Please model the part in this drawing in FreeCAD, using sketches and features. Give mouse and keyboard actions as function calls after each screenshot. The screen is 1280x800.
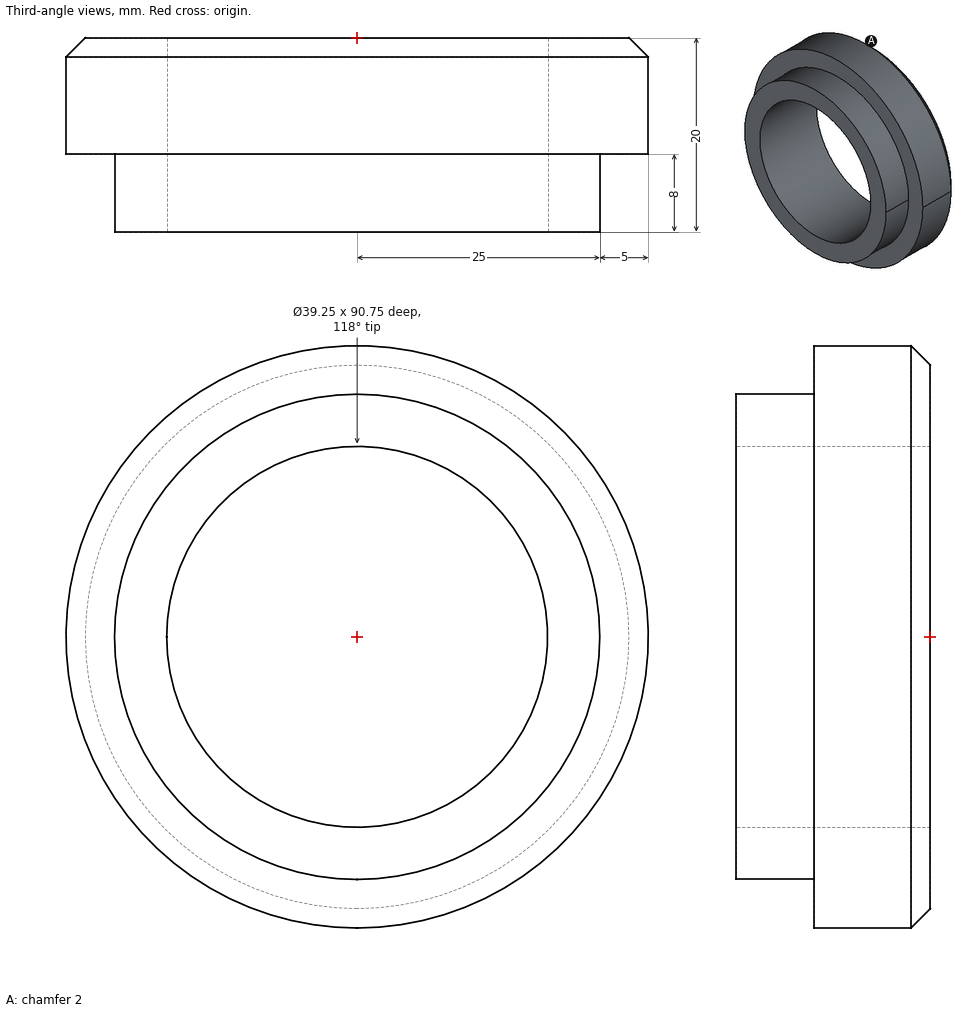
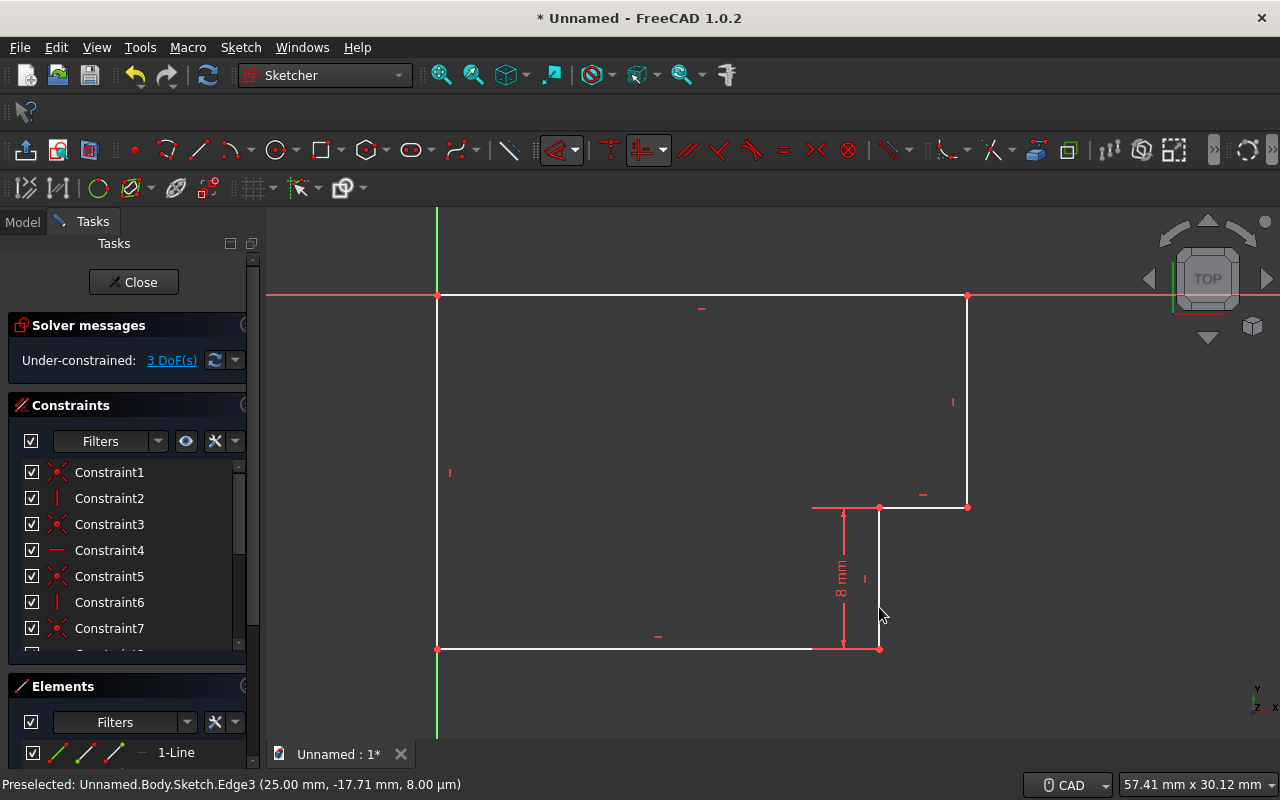
click(905, 508)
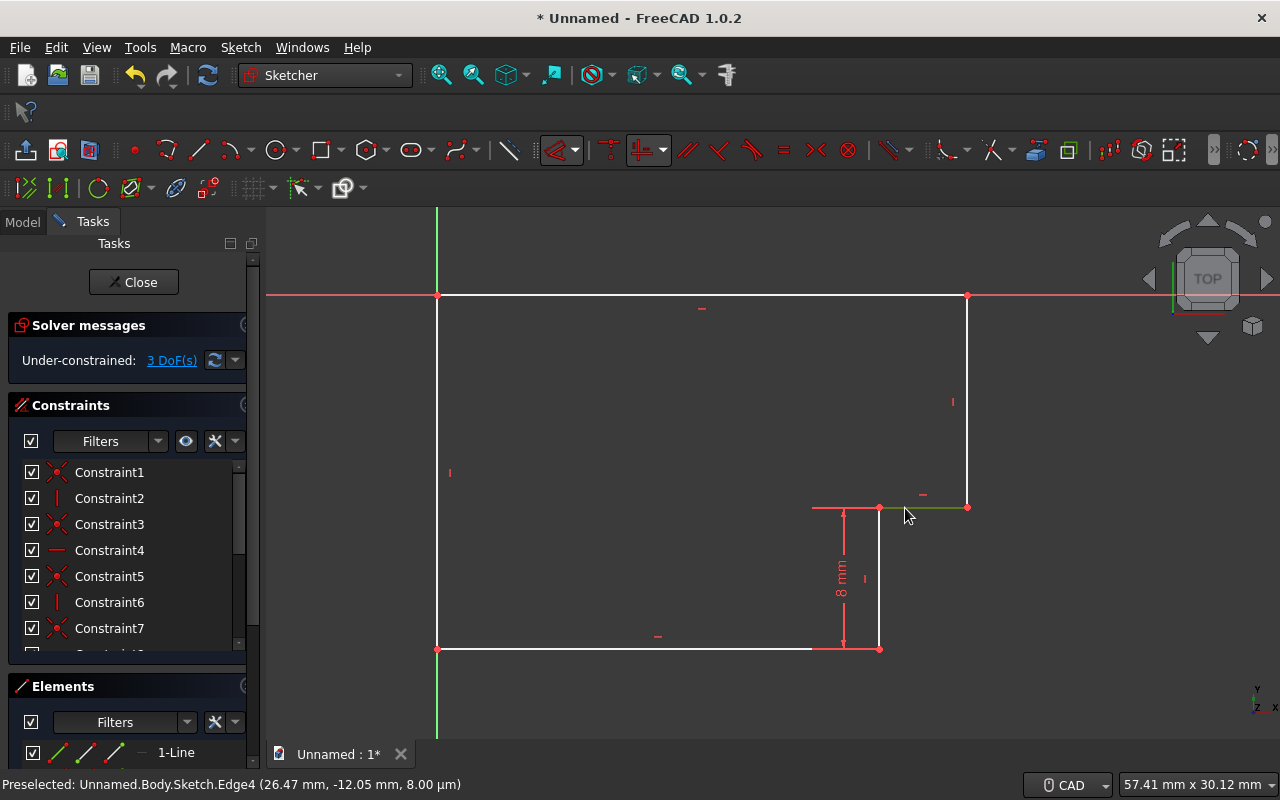
key(l)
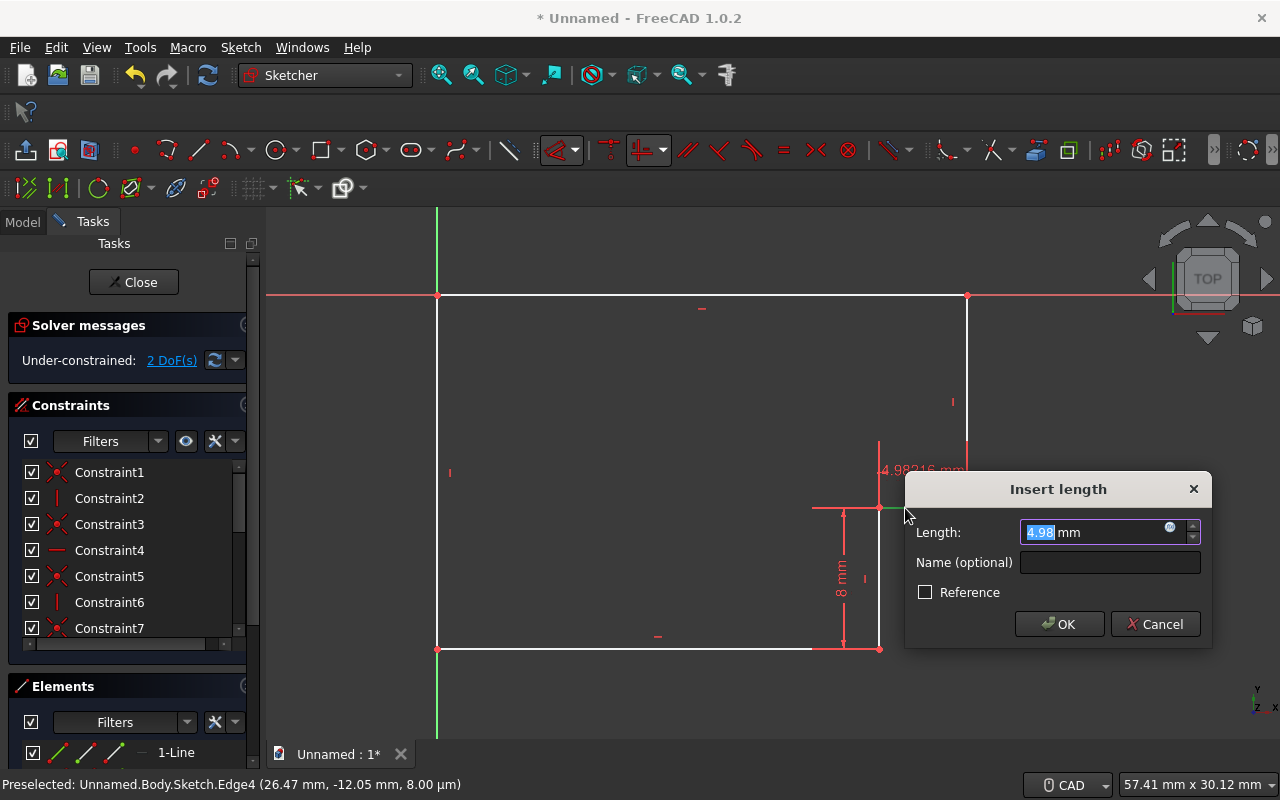
text(5)
key(Return)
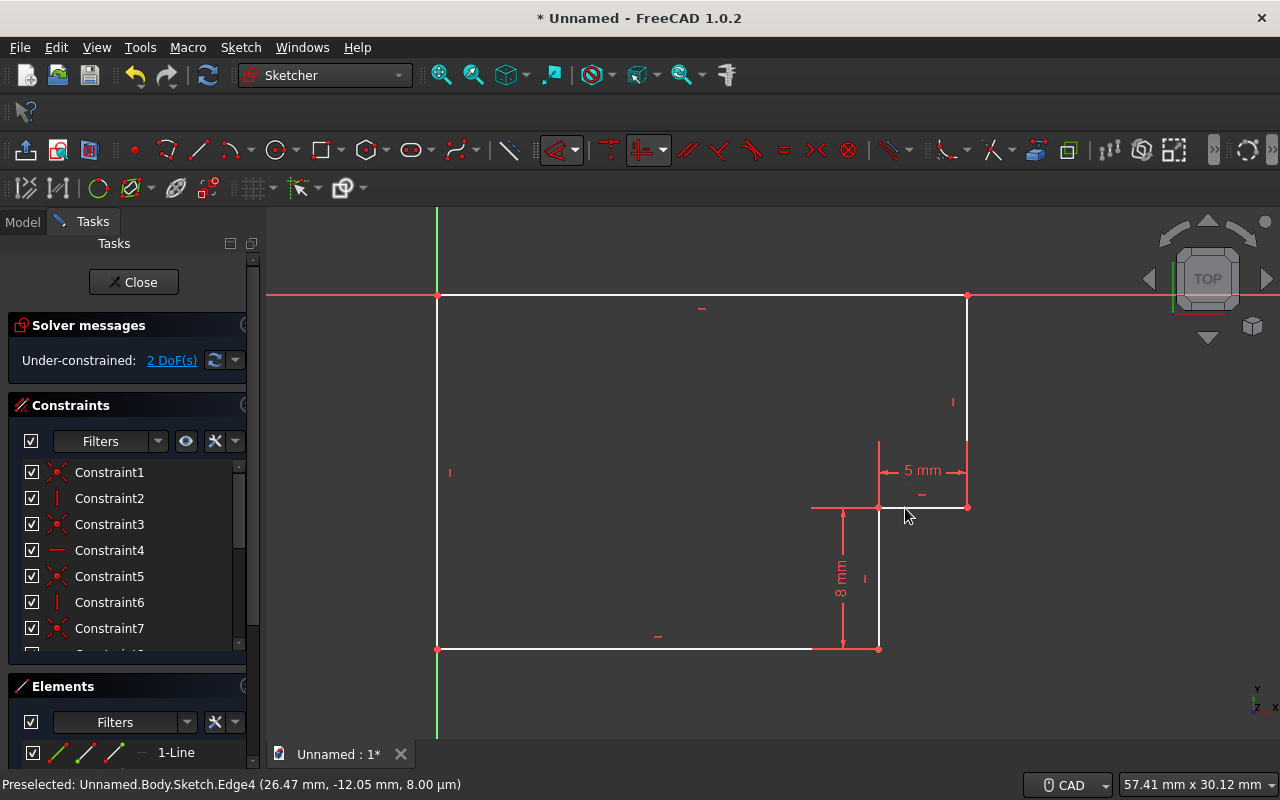
click(437, 401)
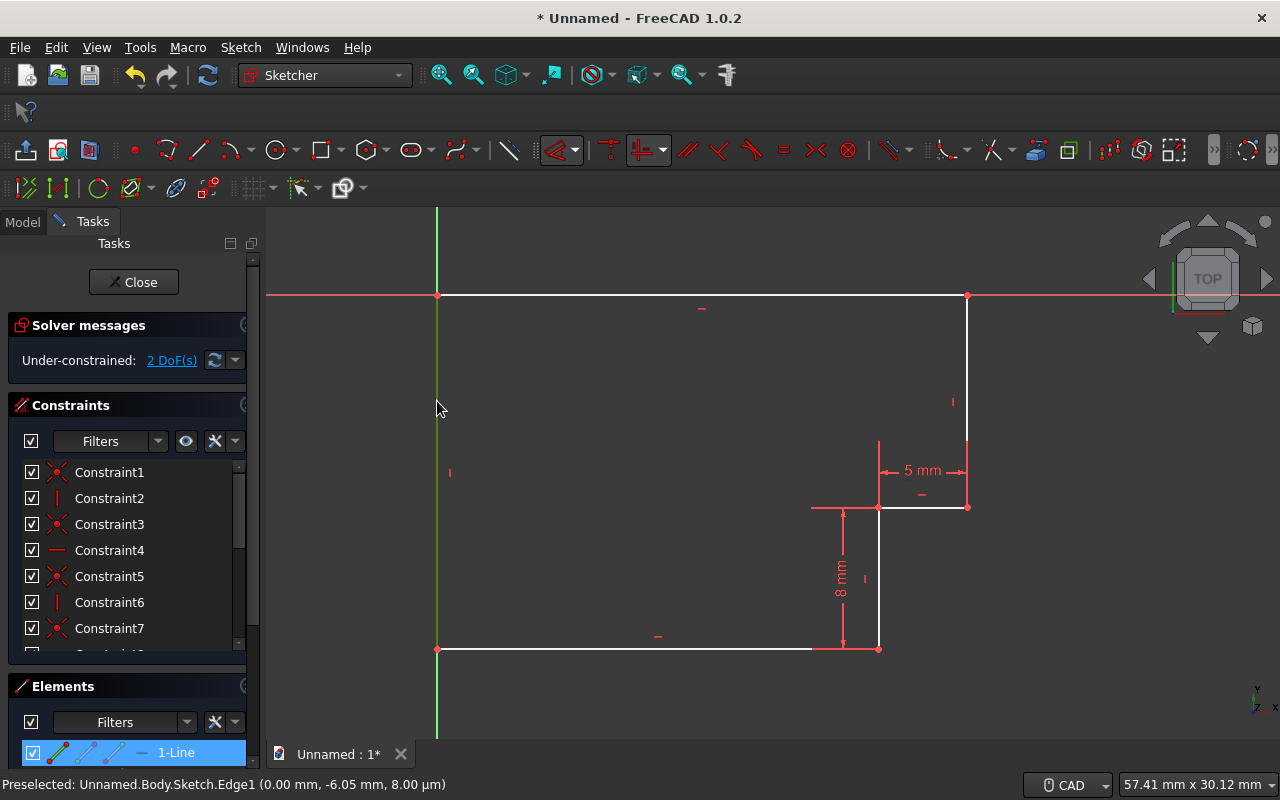
click(578, 150)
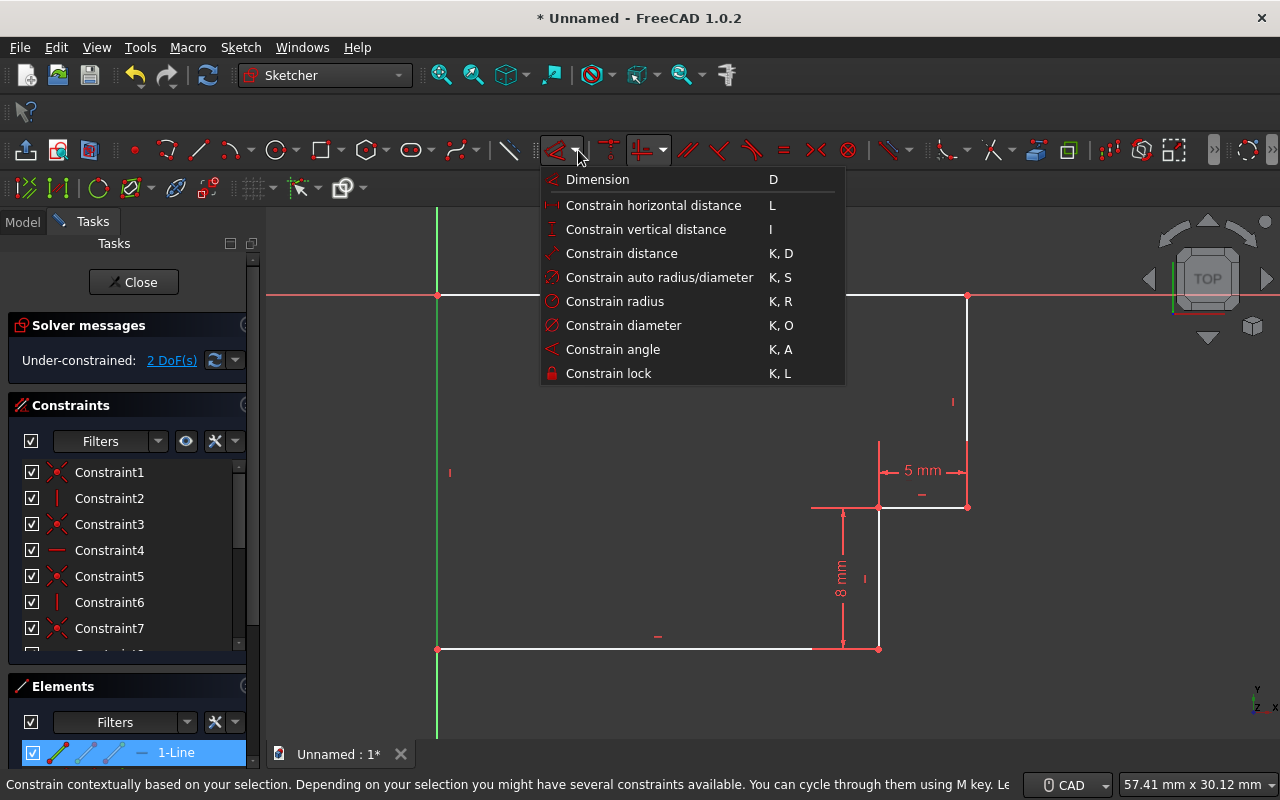
click(693, 229)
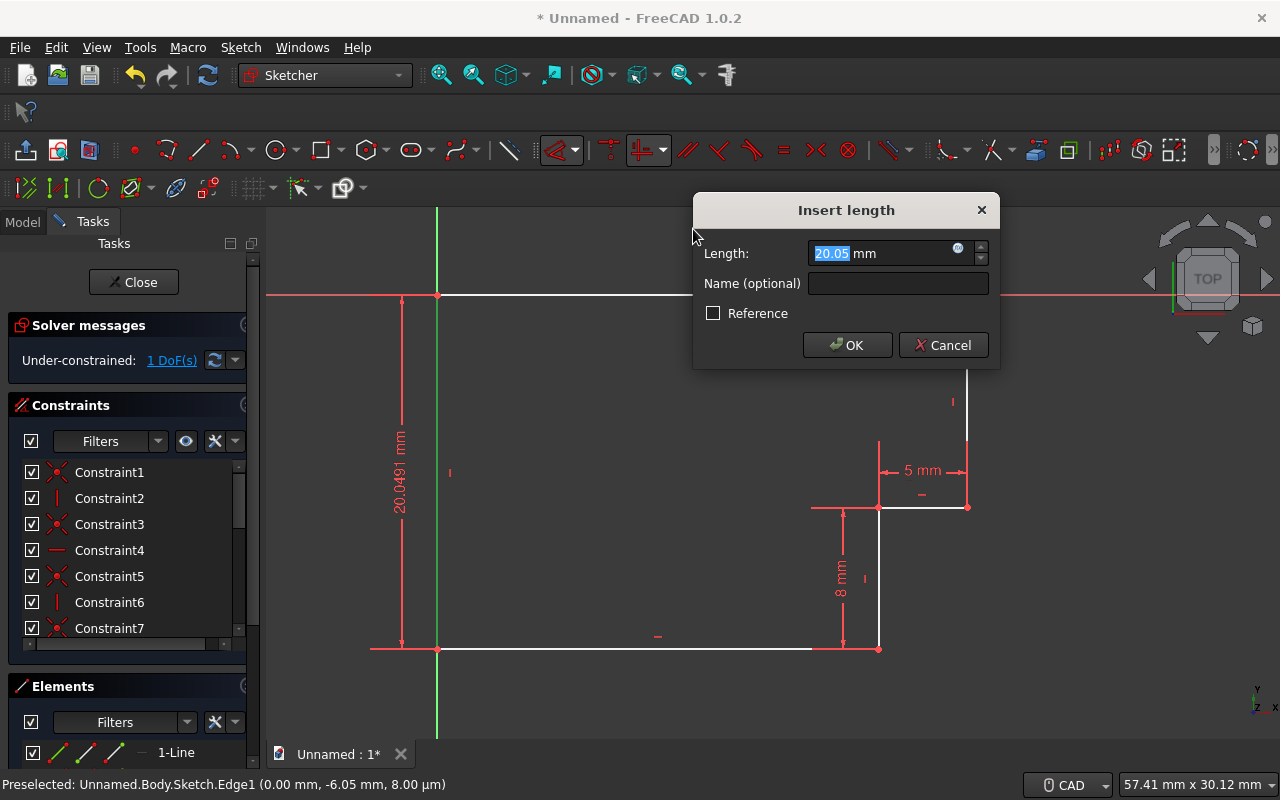
text(20)
key(Return)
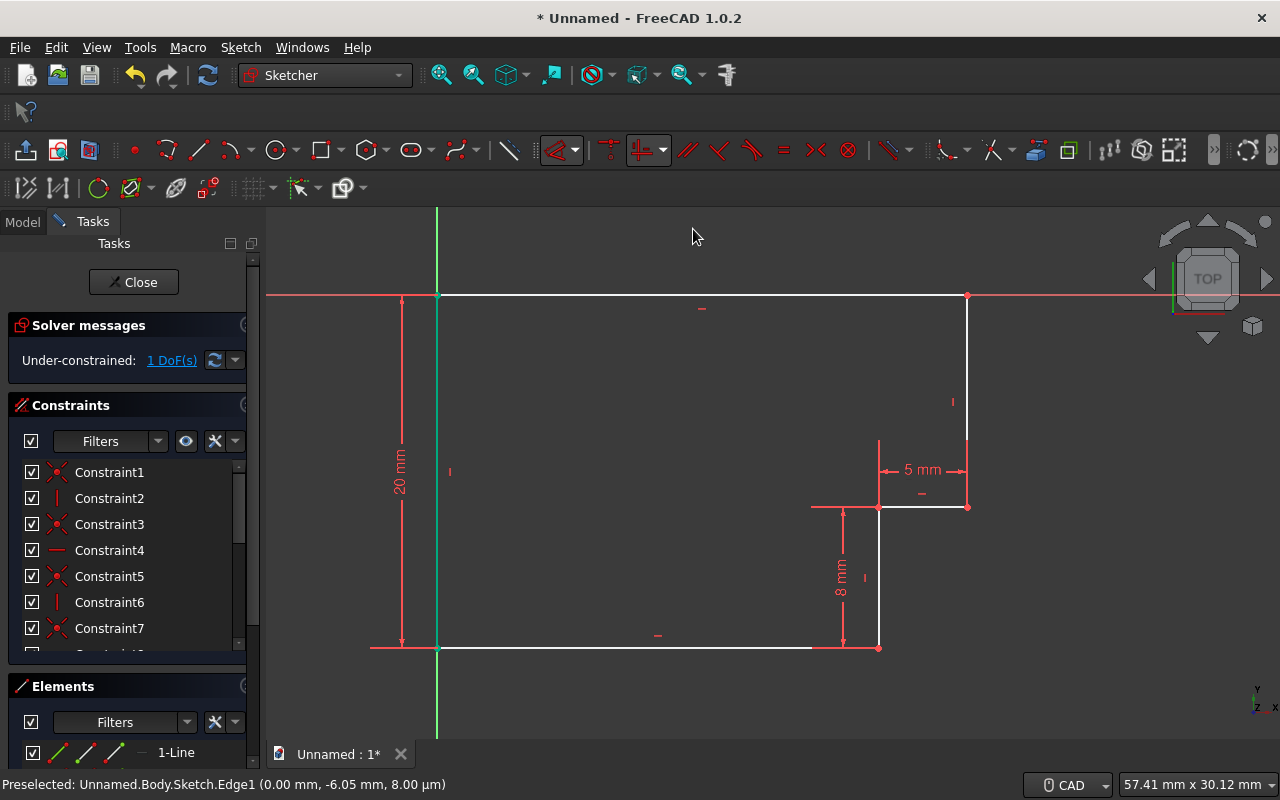
click(570, 648)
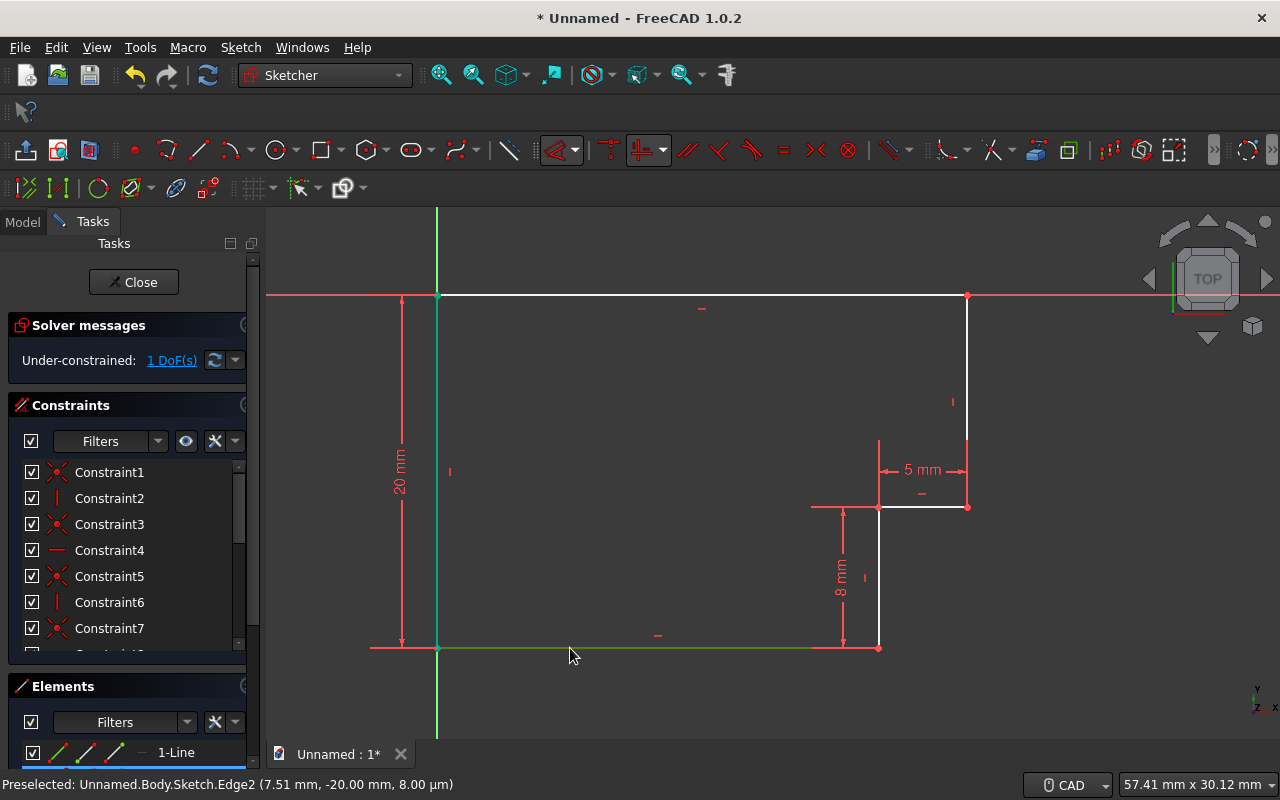
click(578, 150)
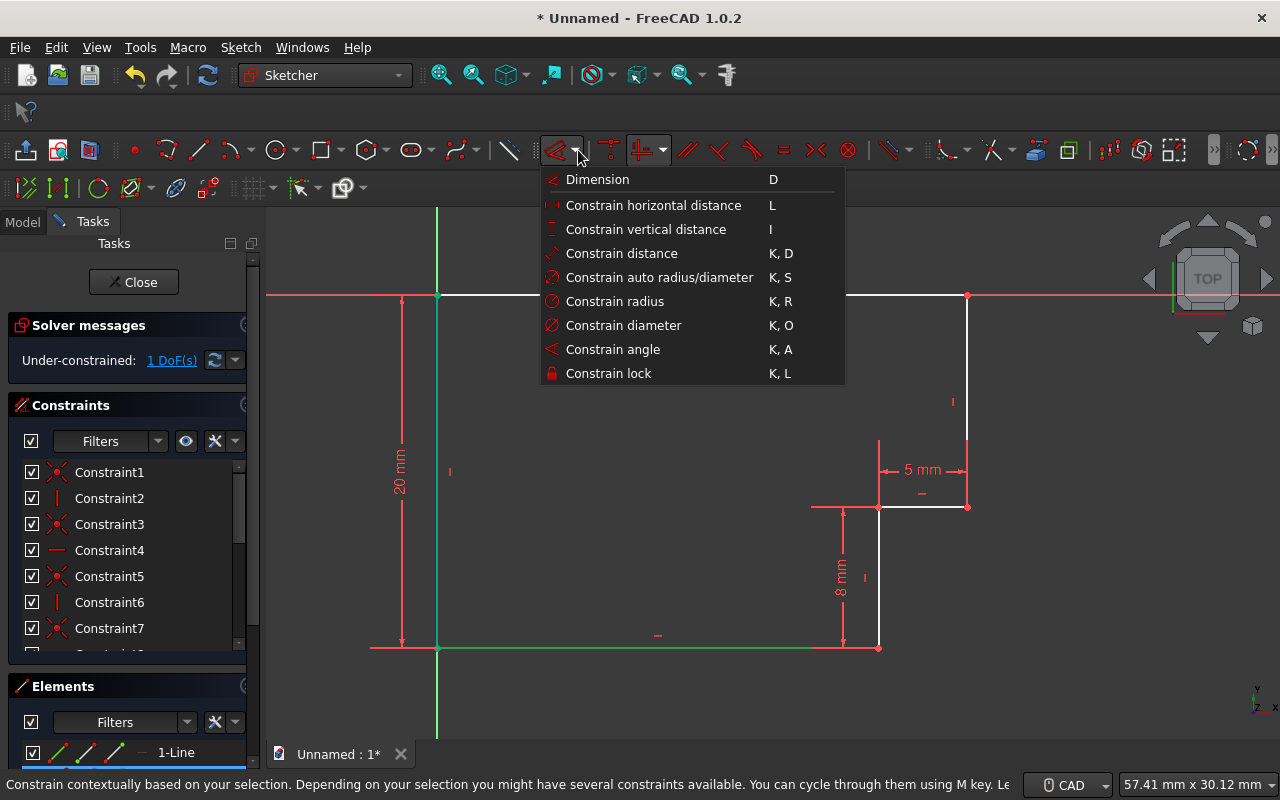
click(693, 205)